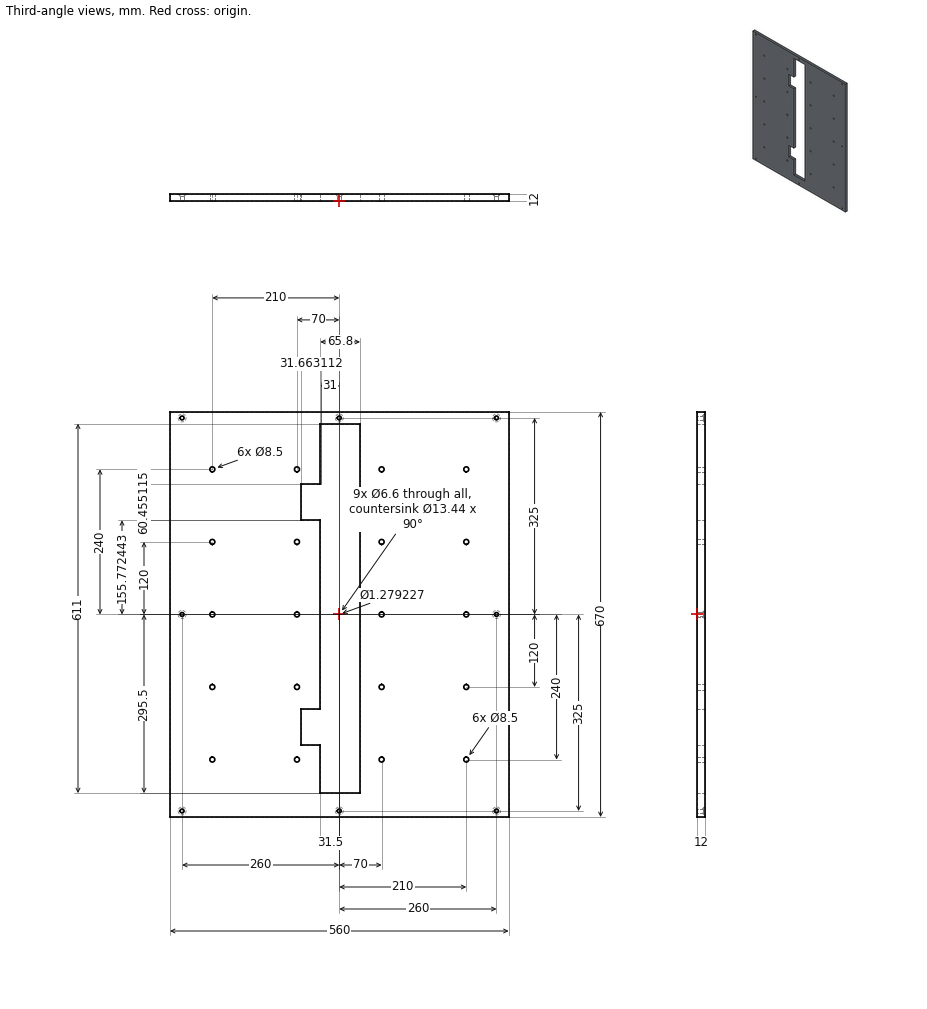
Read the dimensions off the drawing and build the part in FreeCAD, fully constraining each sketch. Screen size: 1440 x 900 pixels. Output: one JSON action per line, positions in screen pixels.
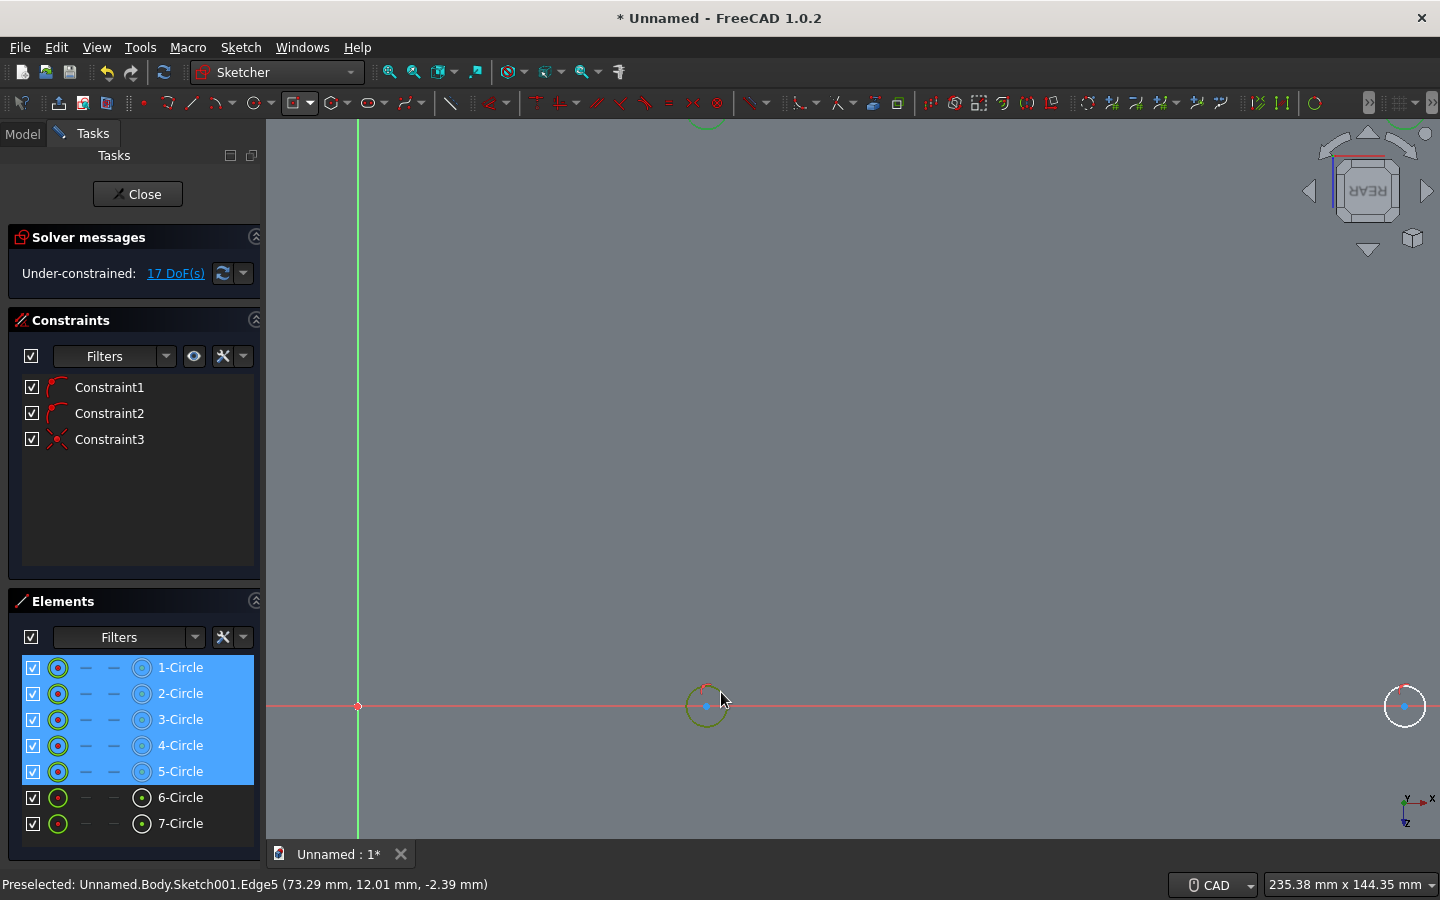
{"action": "scroll", "coordinate": [723, 695], "scroll_direction": "down", "scroll_amount": 5}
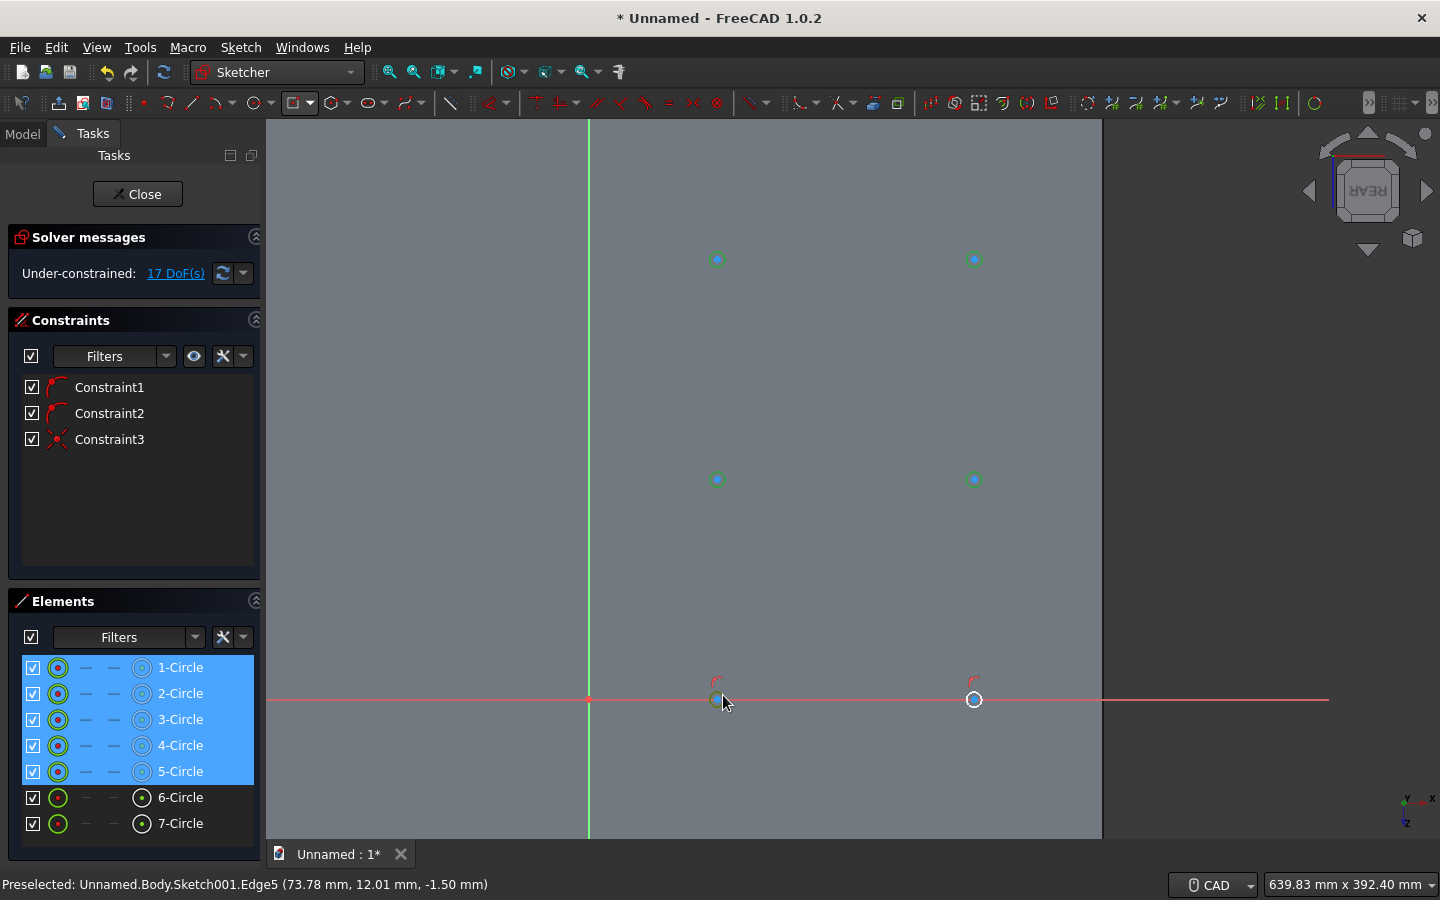
{"action": "scroll", "coordinate": [979, 694], "scroll_direction": "up", "scroll_amount": 5}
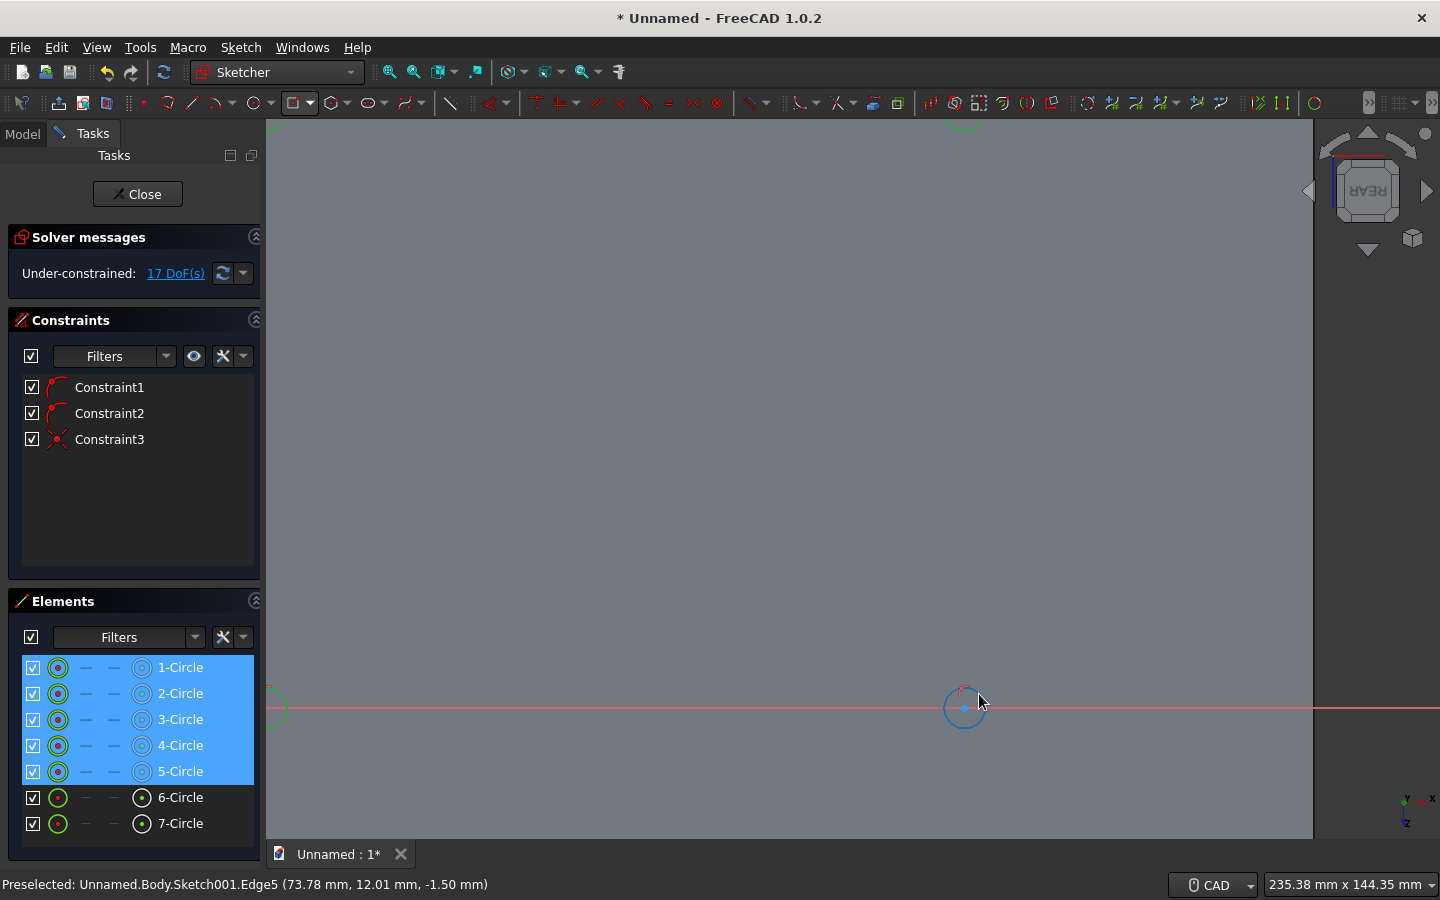
{"action": "left_click", "coordinate": [979, 694]}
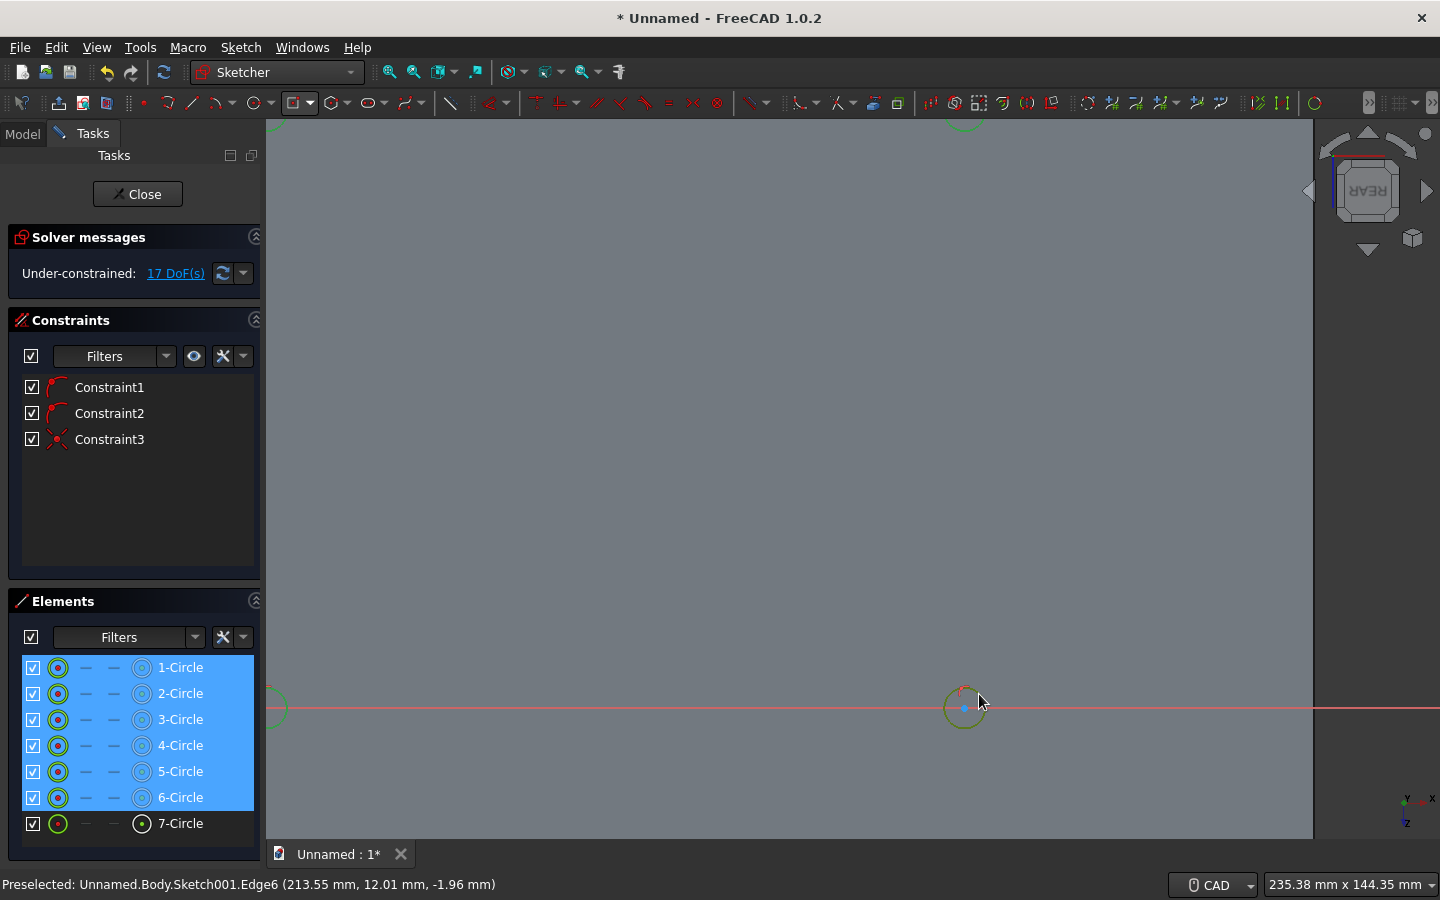
{"action": "left_click", "coordinate": [670, 104]}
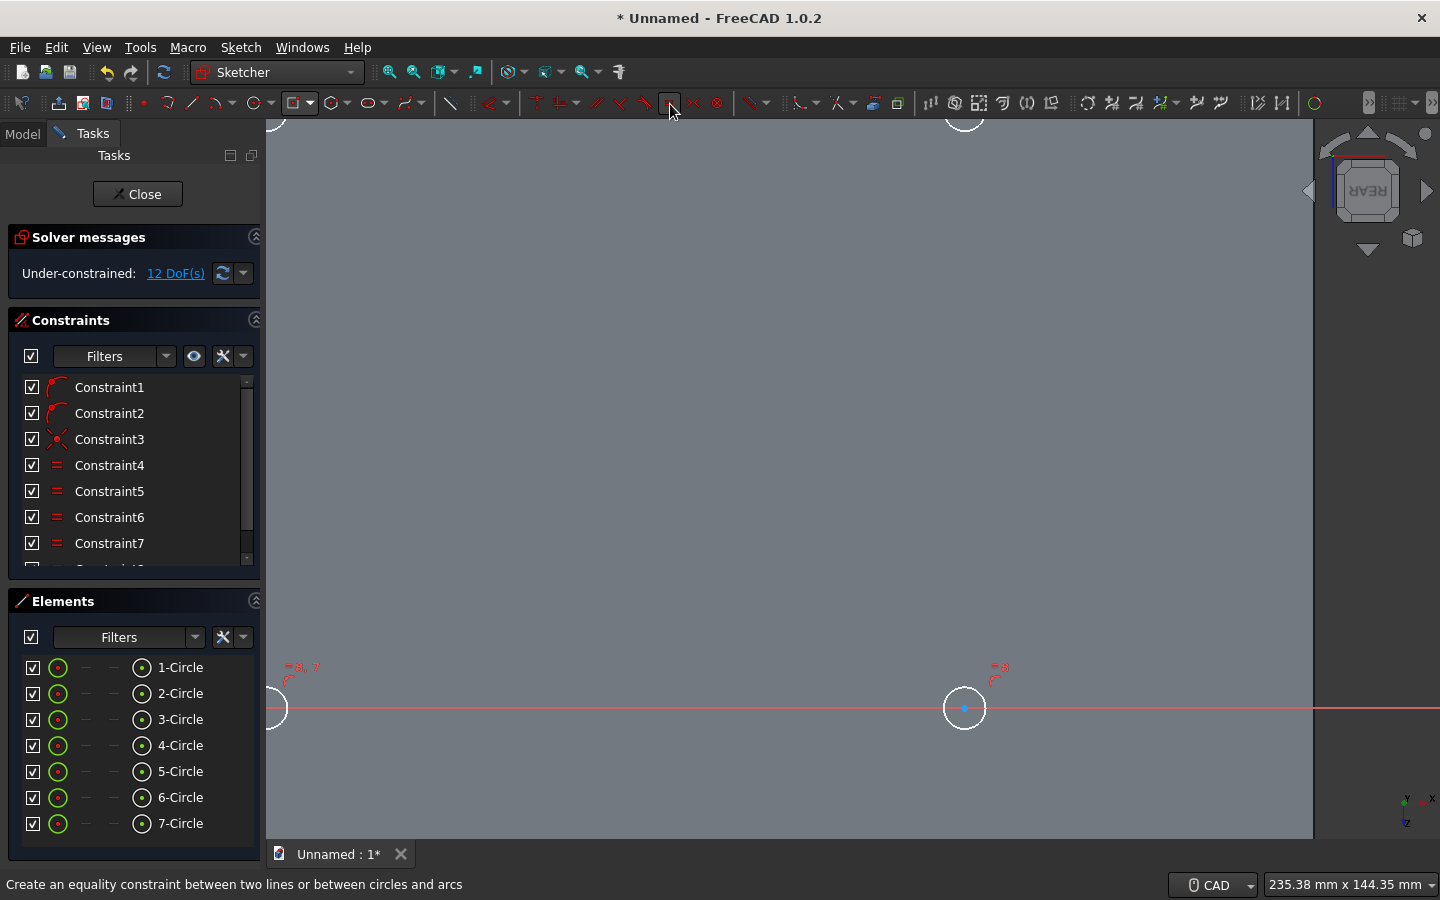
{"action": "scroll", "coordinate": [979, 694], "scroll_direction": "down", "scroll_amount": 5}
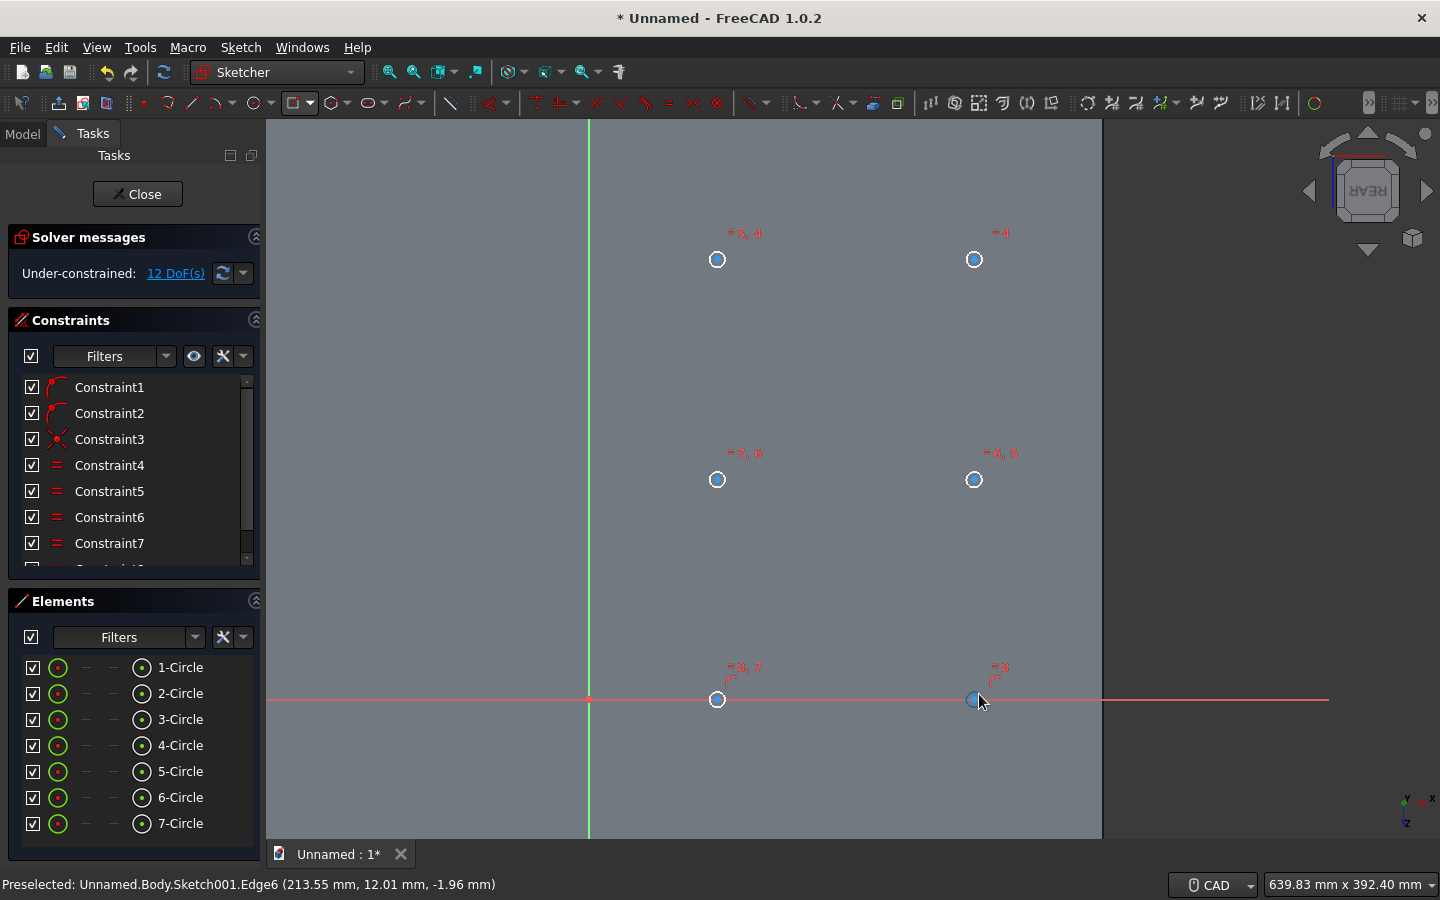
{"action": "left_click", "coordinate": [974, 260]}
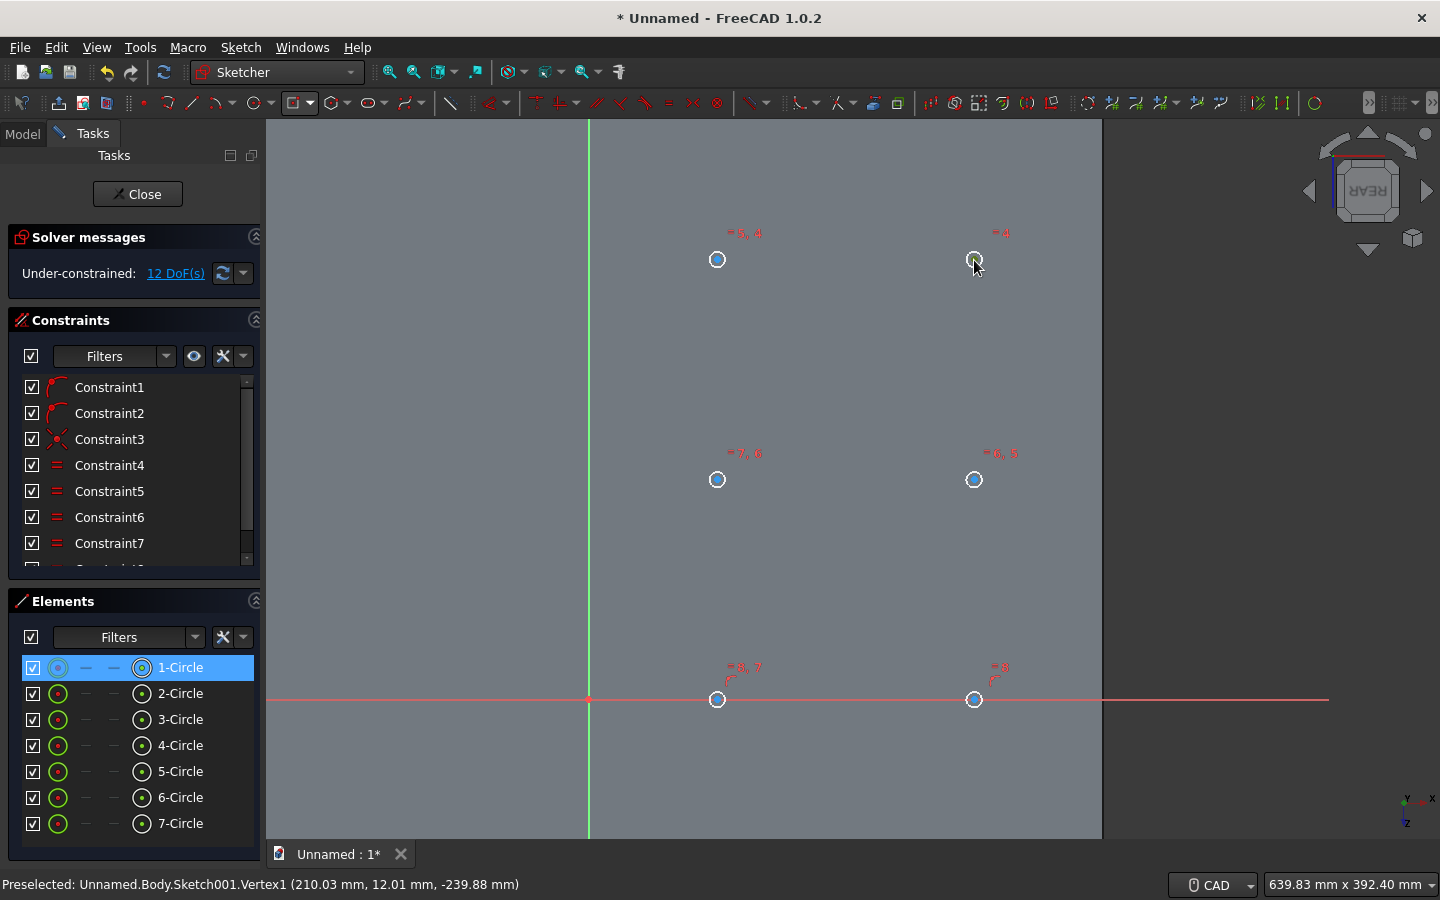
{"action": "left_click", "coordinate": [717, 260]}